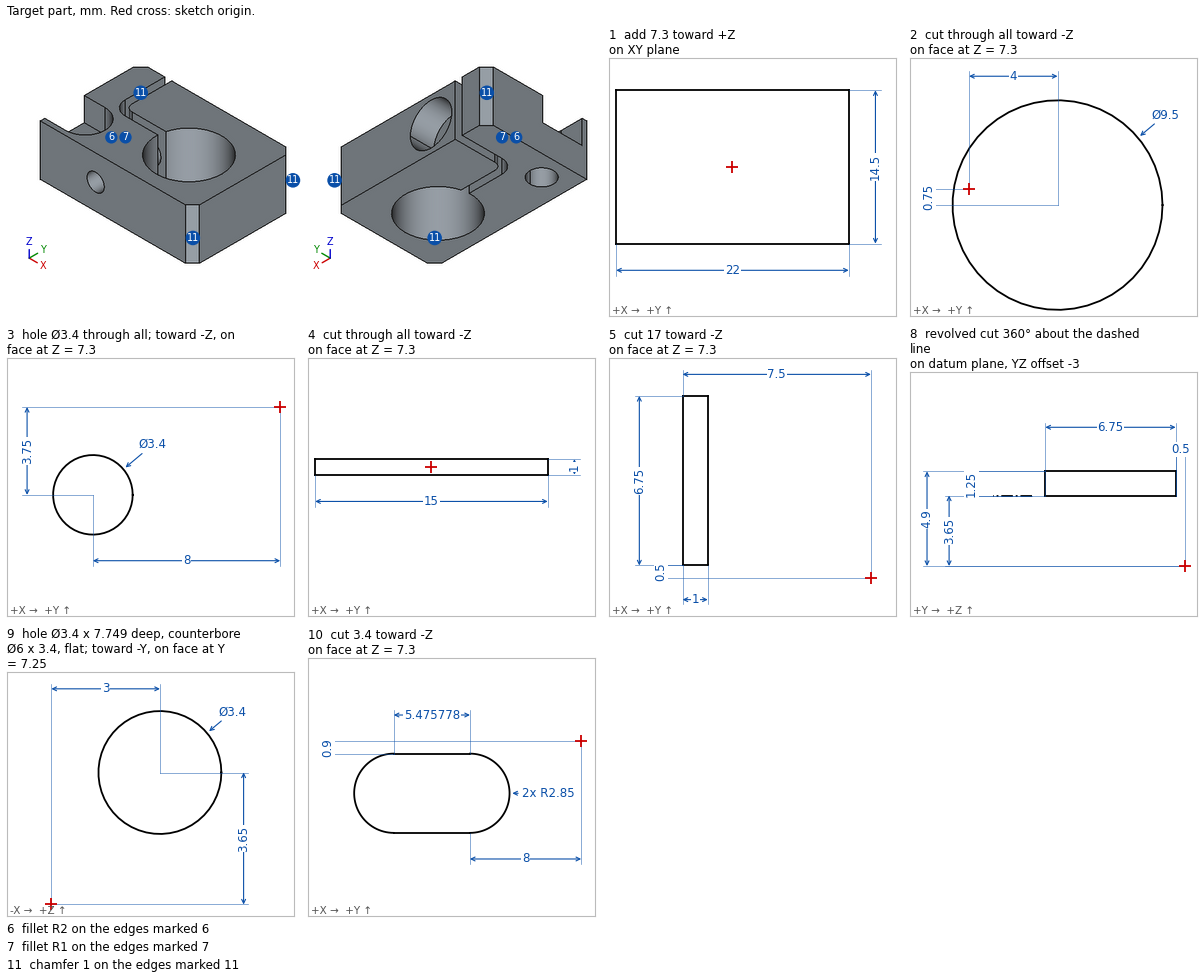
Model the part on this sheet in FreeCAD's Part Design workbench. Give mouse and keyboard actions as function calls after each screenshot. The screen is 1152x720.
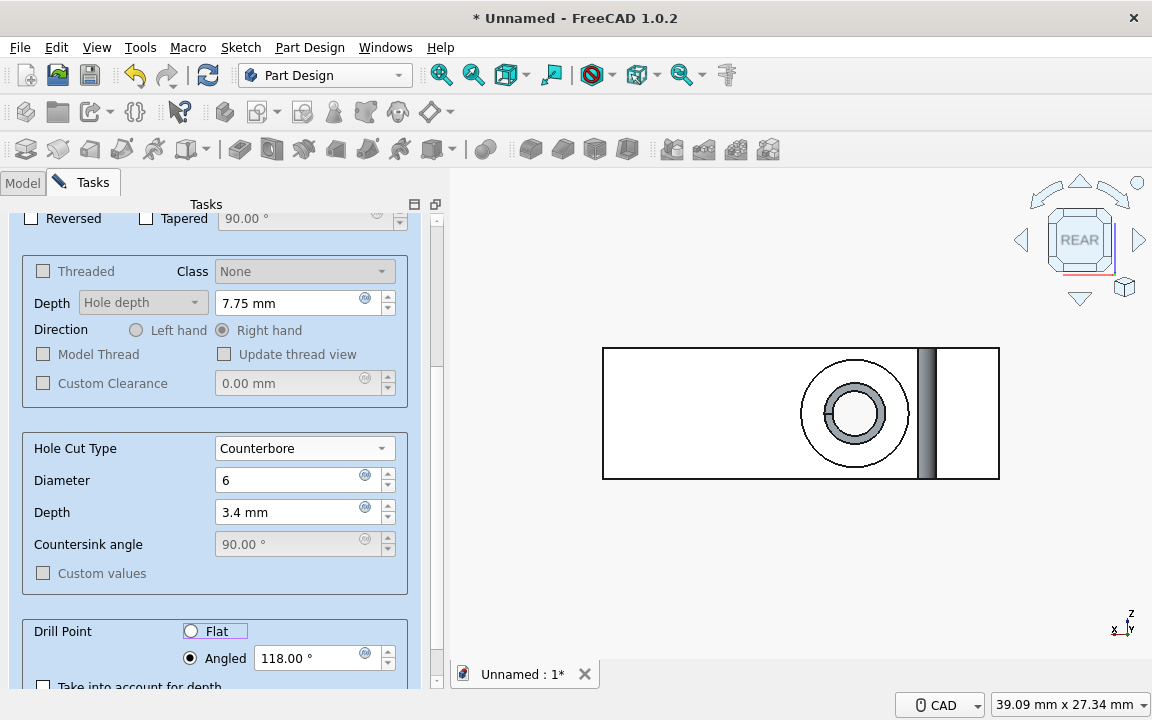
click(191, 631)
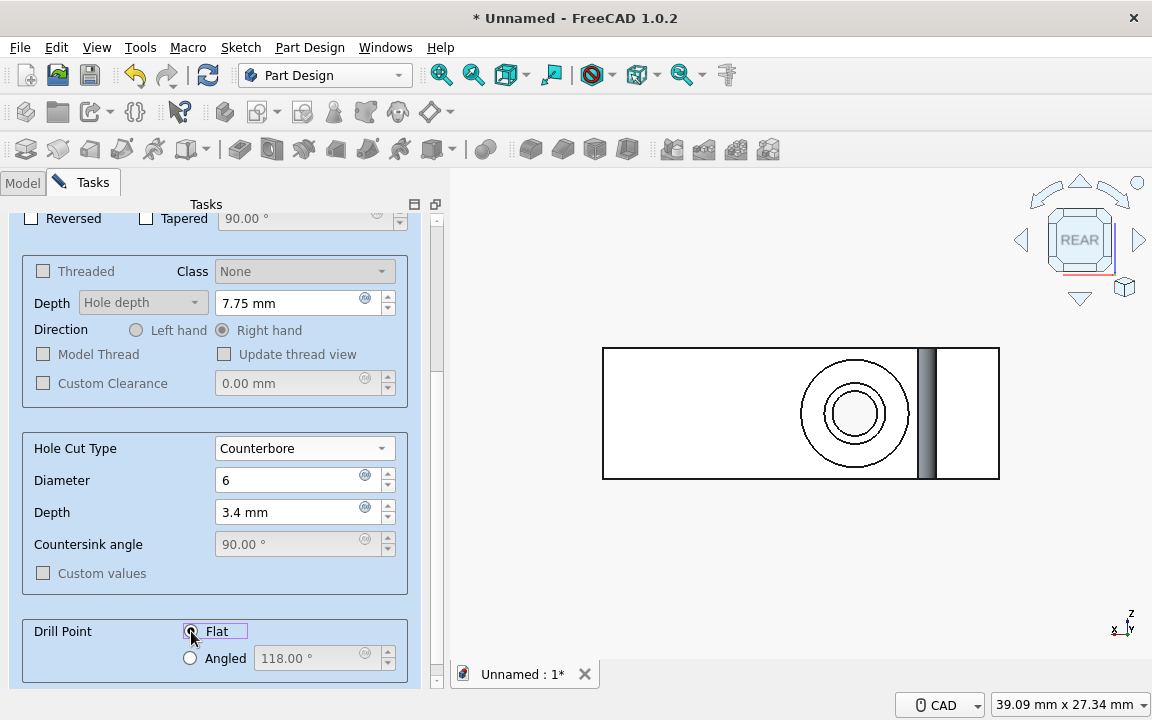
scroll(437, 451, up, 5)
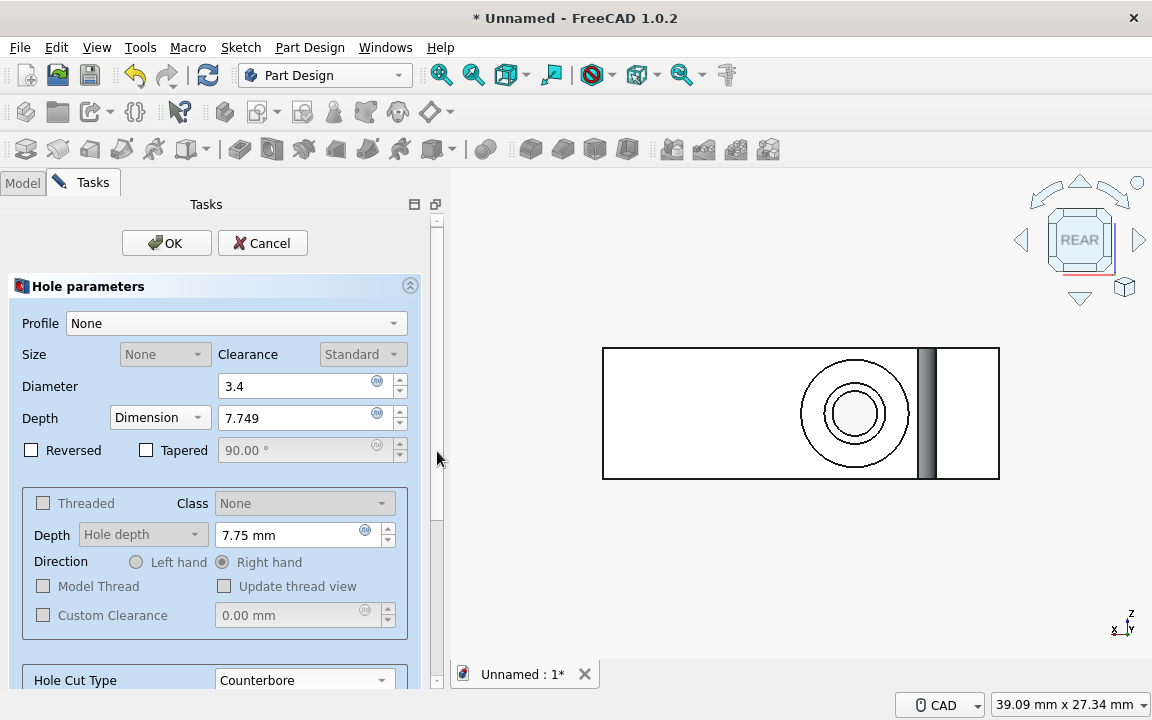
click(167, 243)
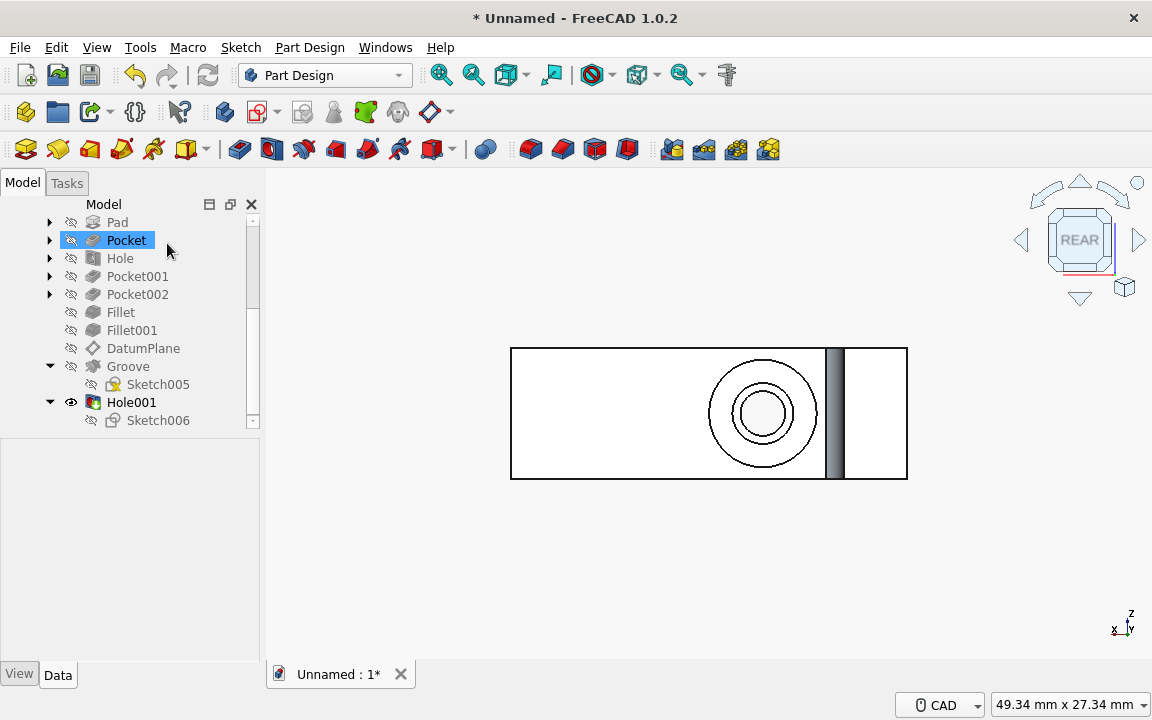
key(v)
key(f)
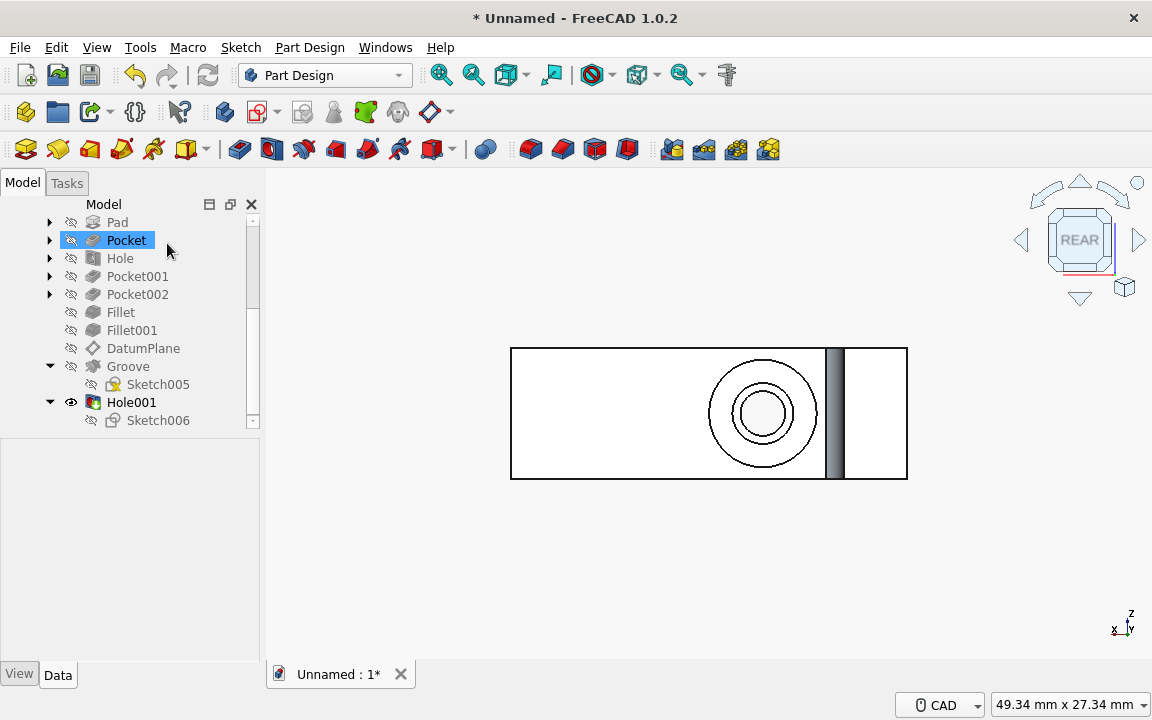
key(0)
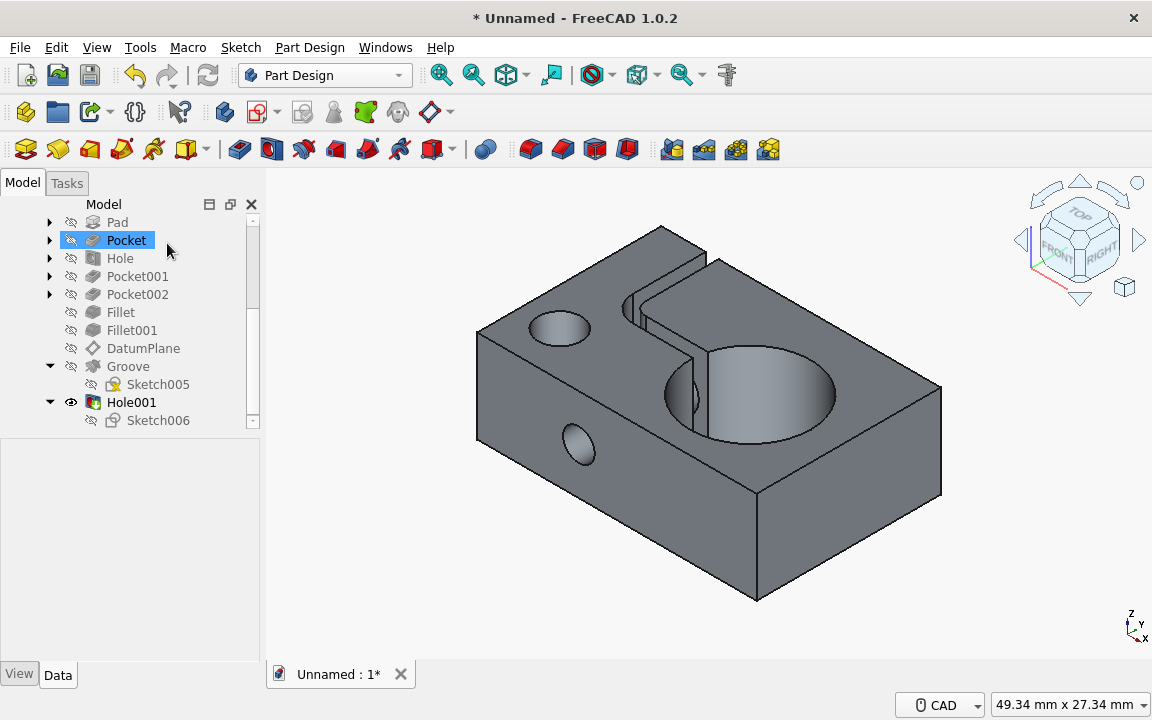
click(722, 306)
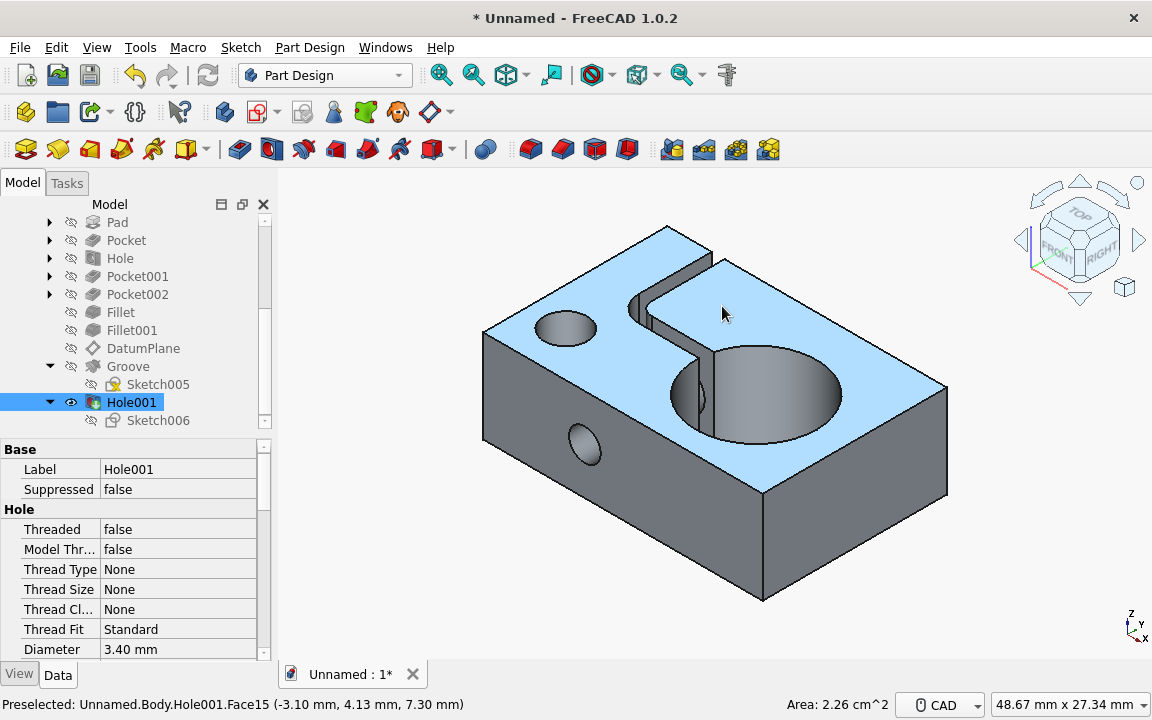
click(258, 112)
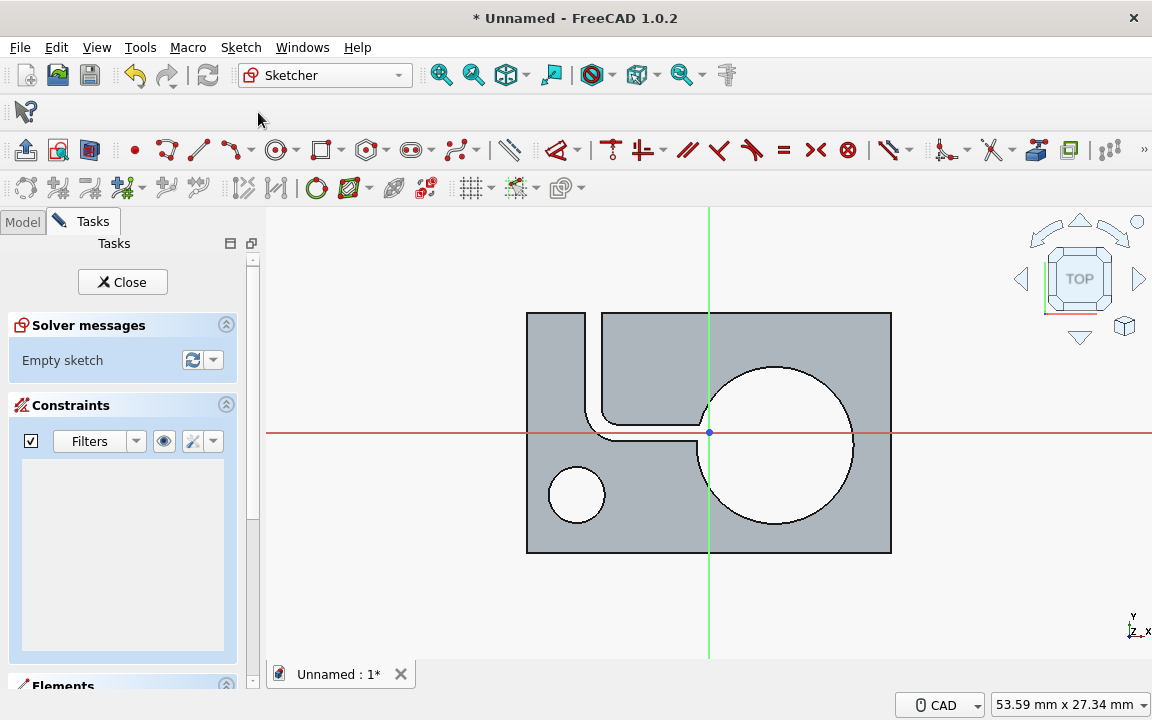
scroll(493, 554, up, 3)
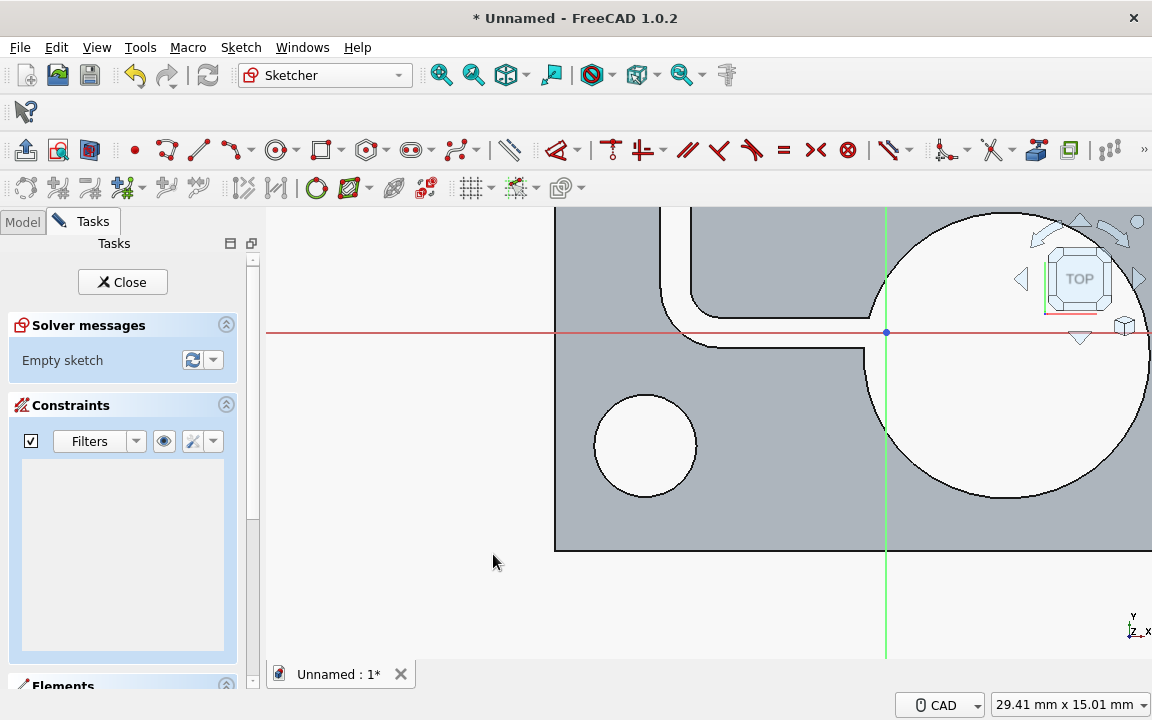
click(412, 150)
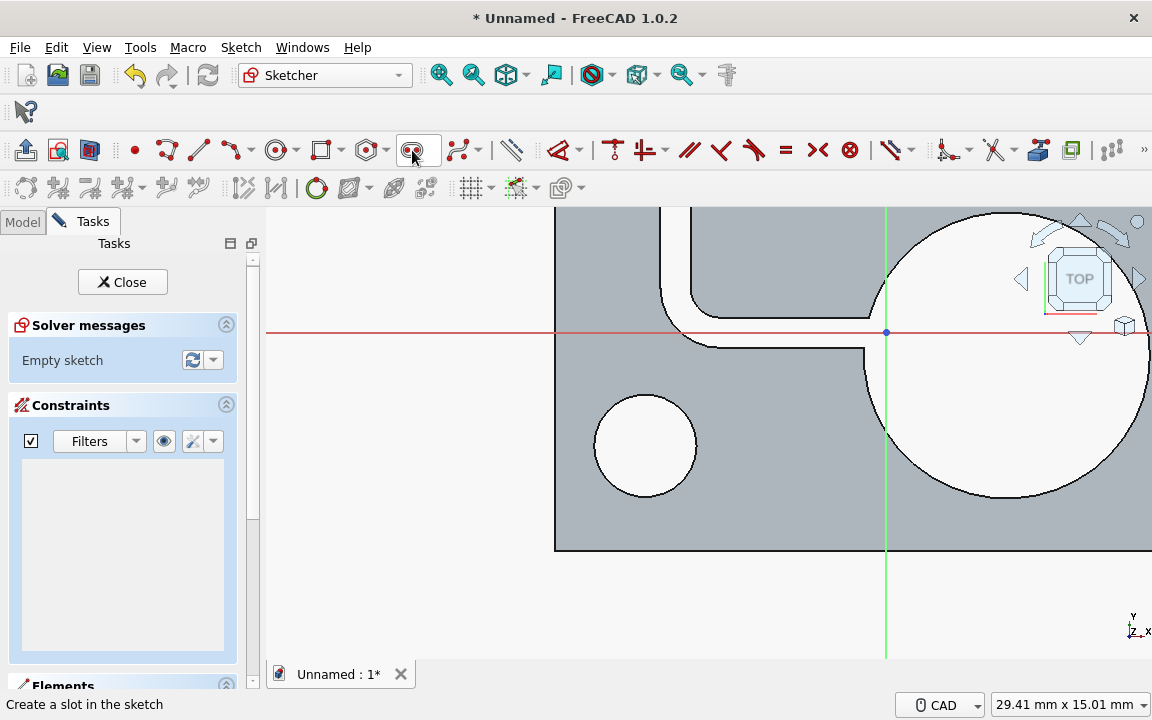
click(480, 446)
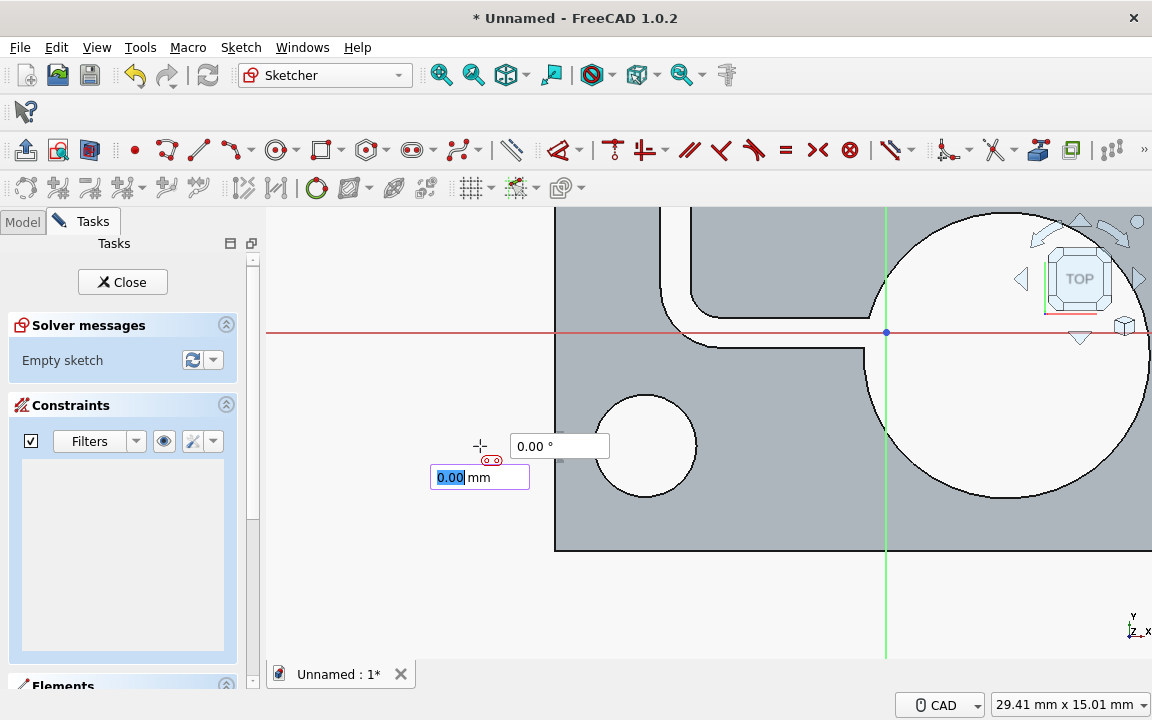
click(645, 446)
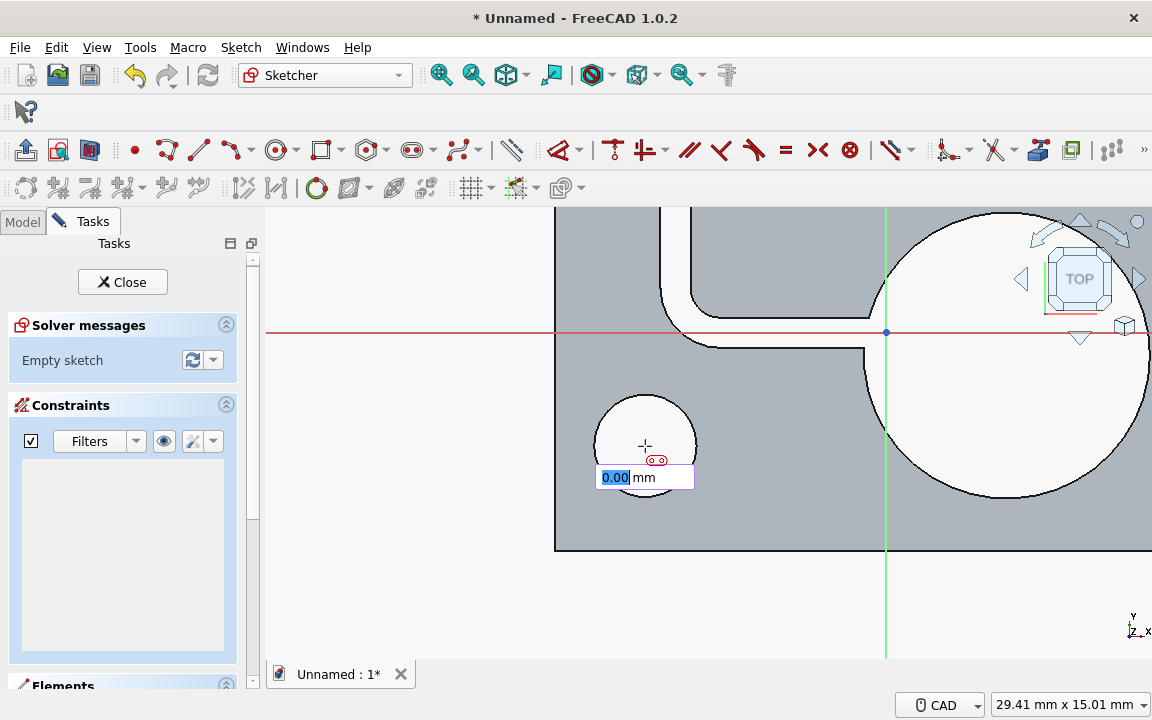
click(563, 532)
key(Escape)